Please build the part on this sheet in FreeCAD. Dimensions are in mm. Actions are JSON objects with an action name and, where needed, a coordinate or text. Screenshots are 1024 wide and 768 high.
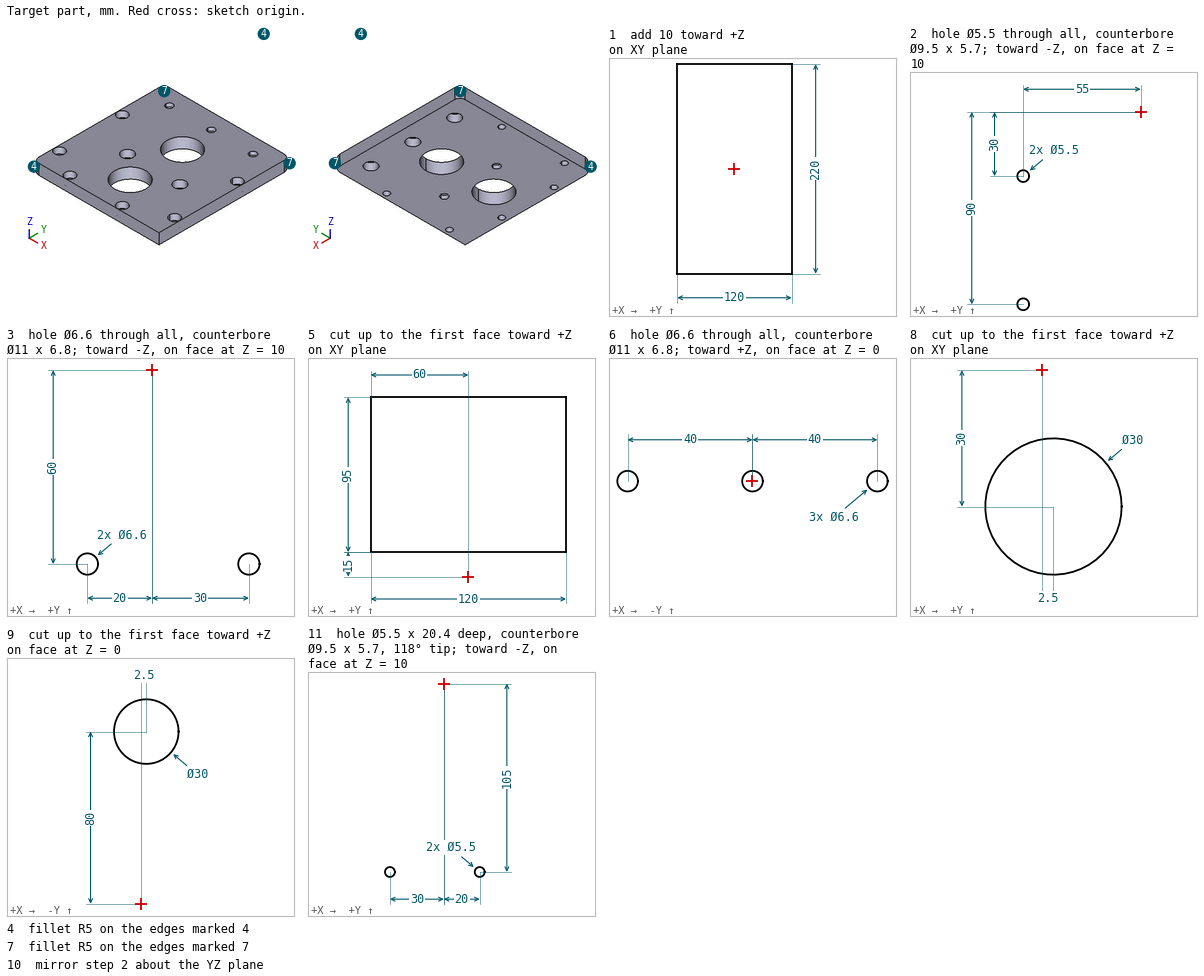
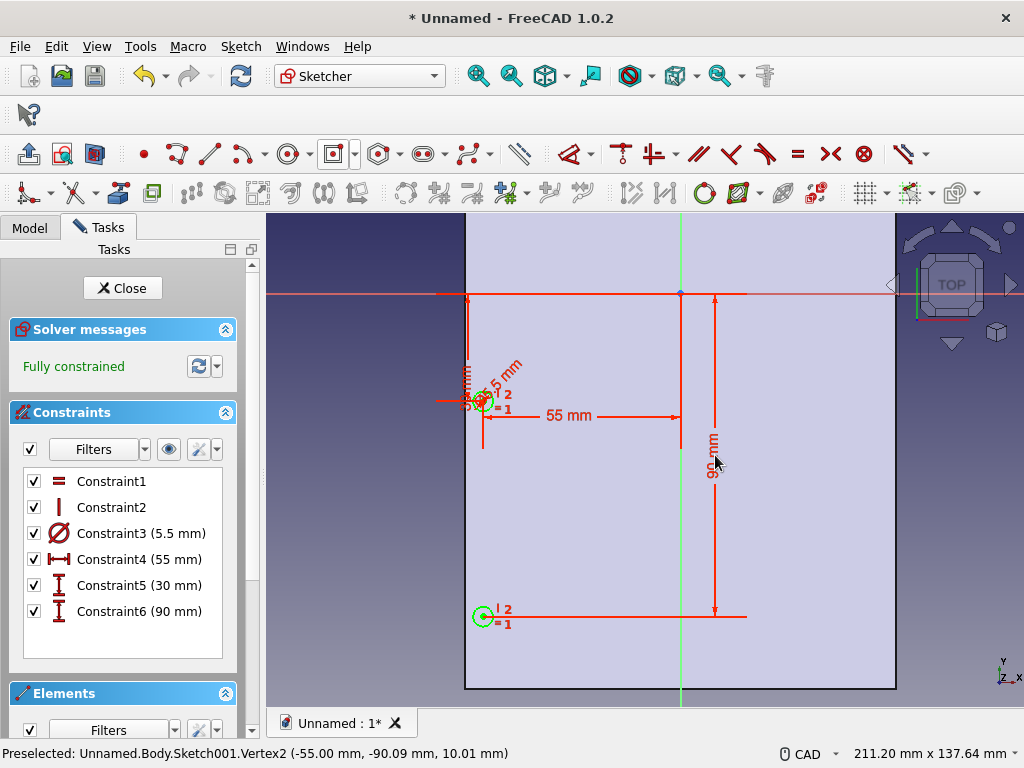
{"action": "left_click", "coordinate": [123, 288]}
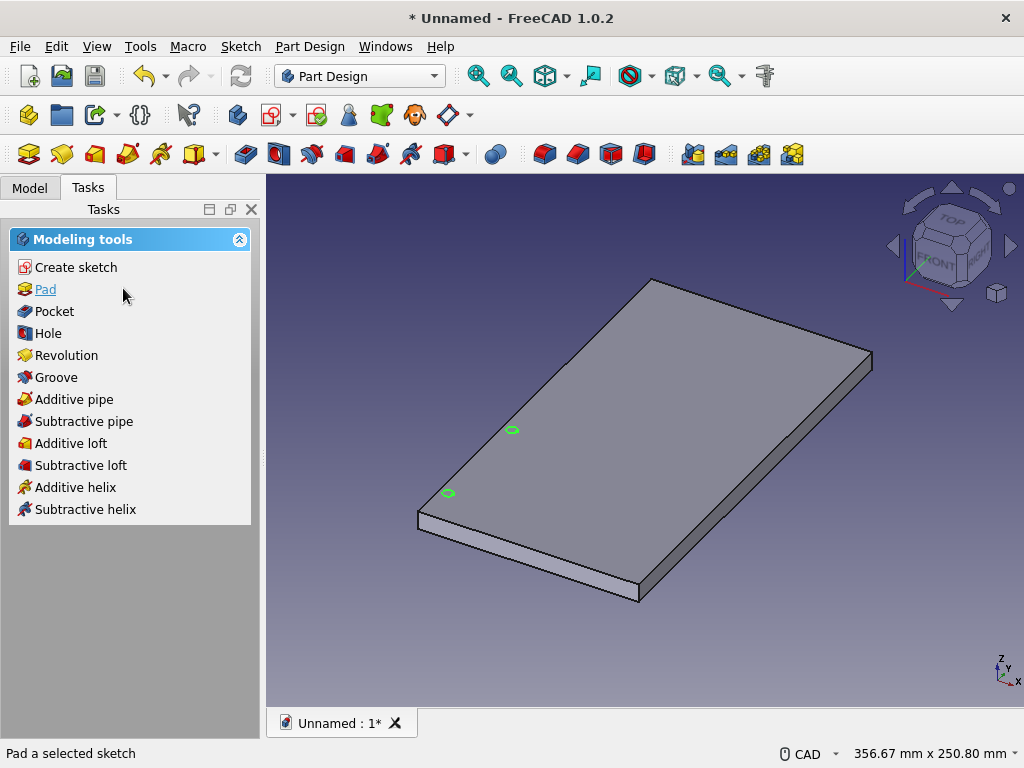
{"action": "left_click", "coordinate": [279, 154]}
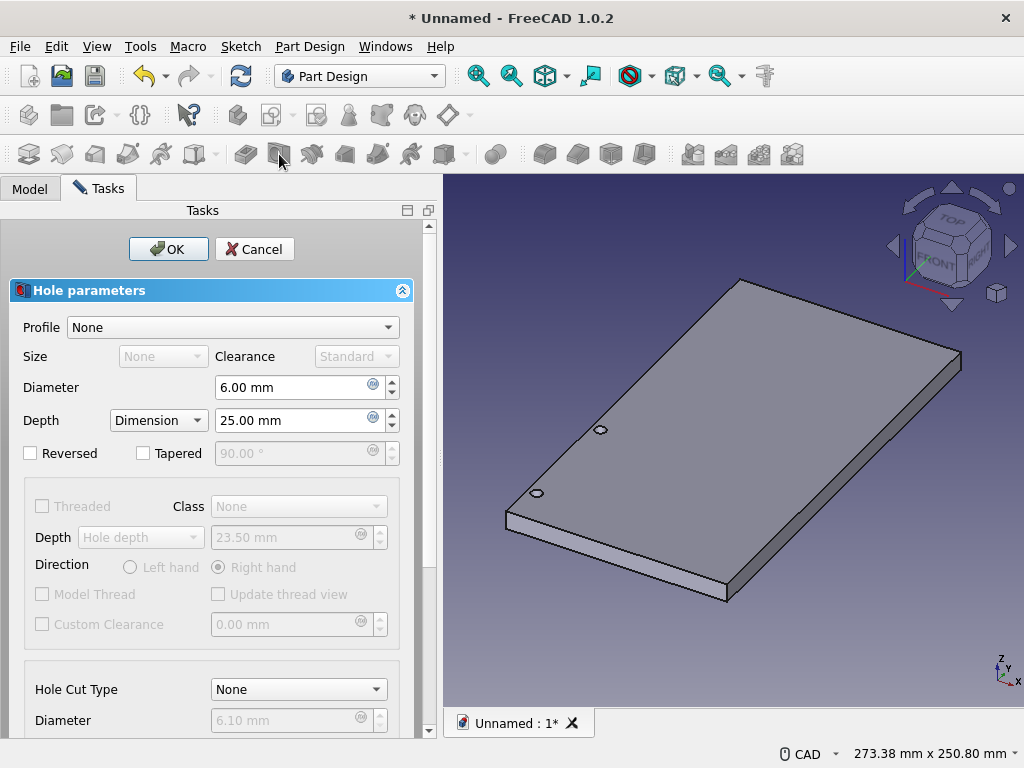
{"action": "triple_click", "coordinate": [300, 388]}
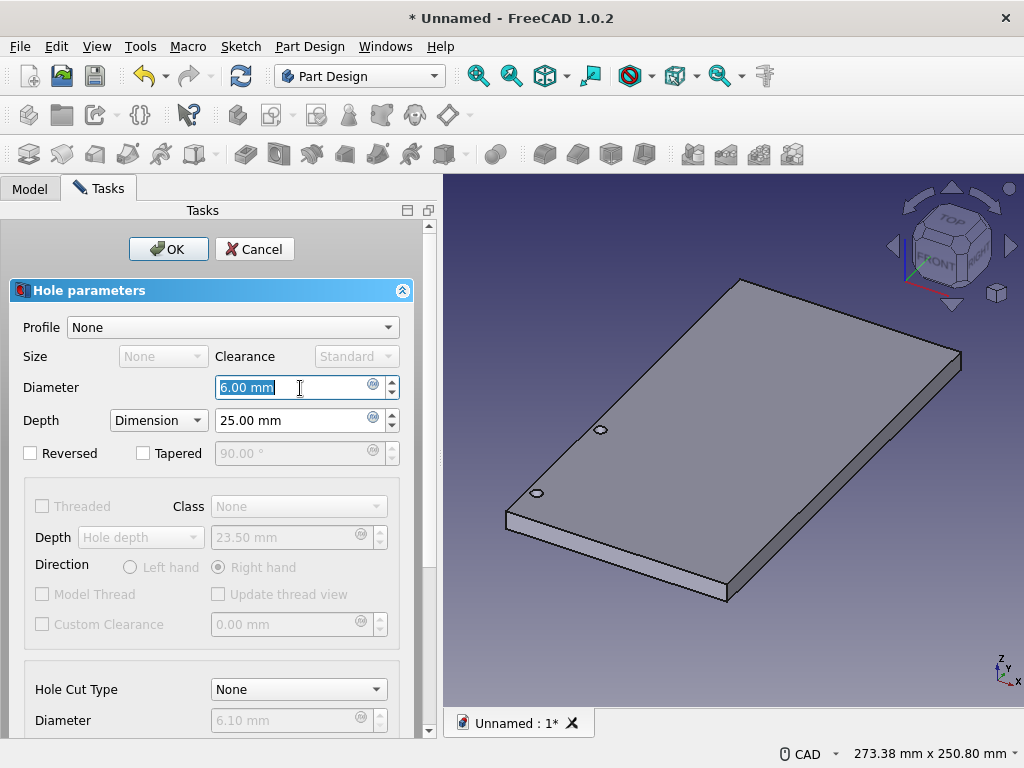
{"action": "type", "text": "5.5"}
{"action": "key", "text": "Tab"}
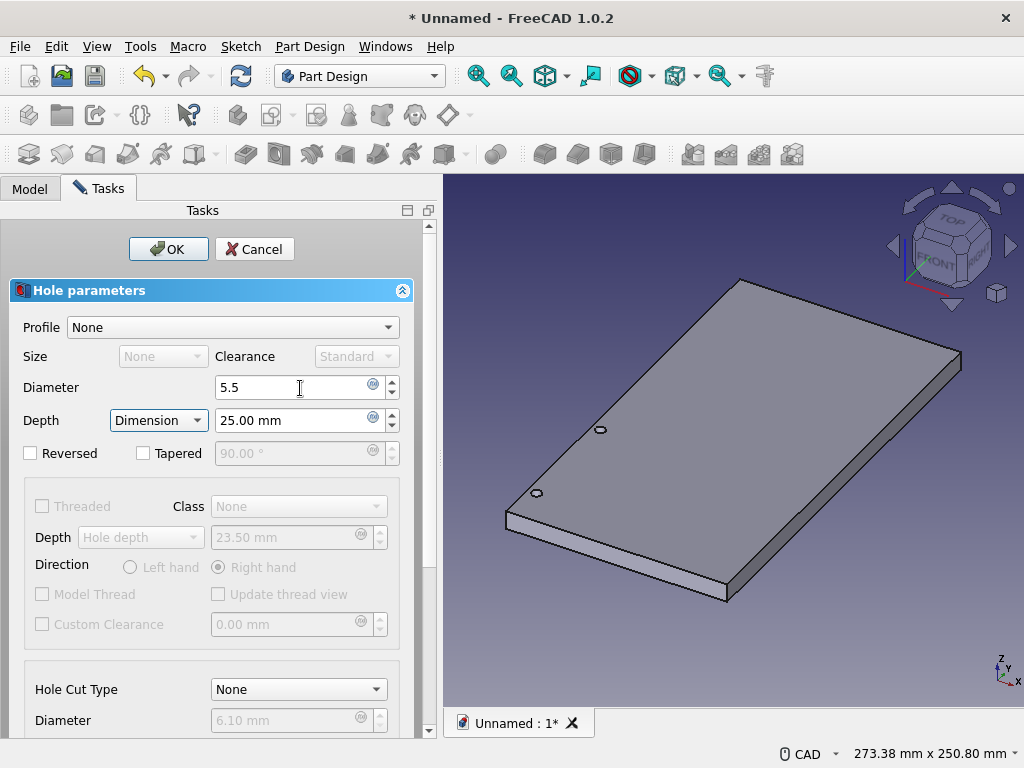
{"action": "left_click", "coordinate": [160, 420]}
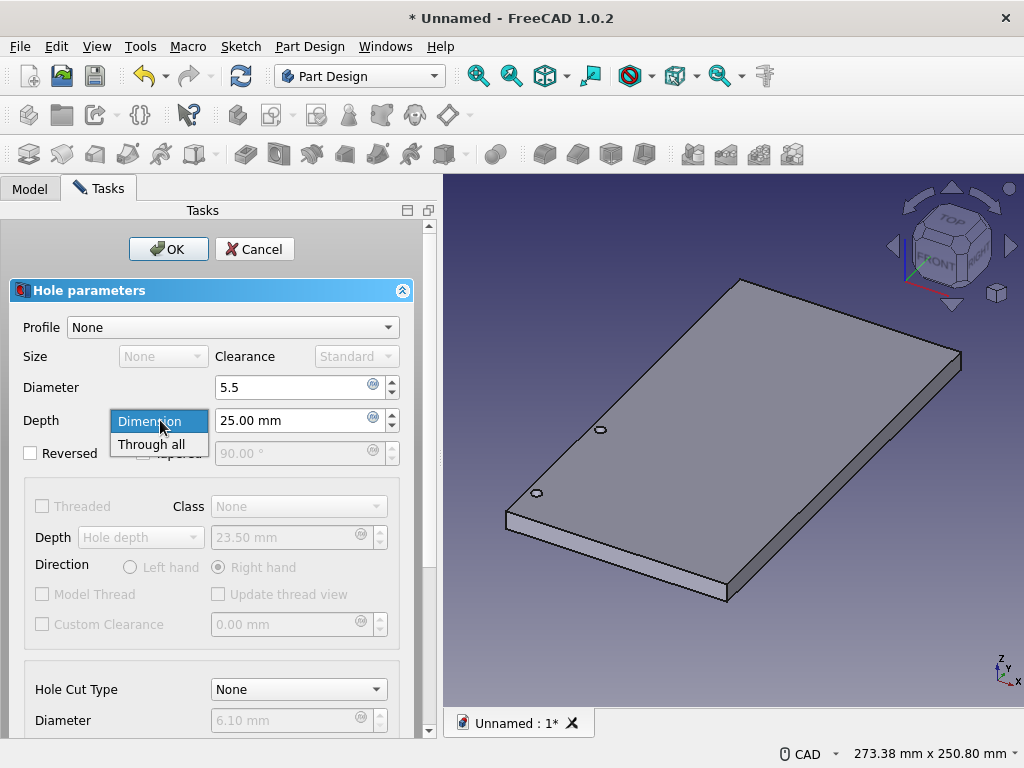
{"action": "left_click", "coordinate": [158, 444]}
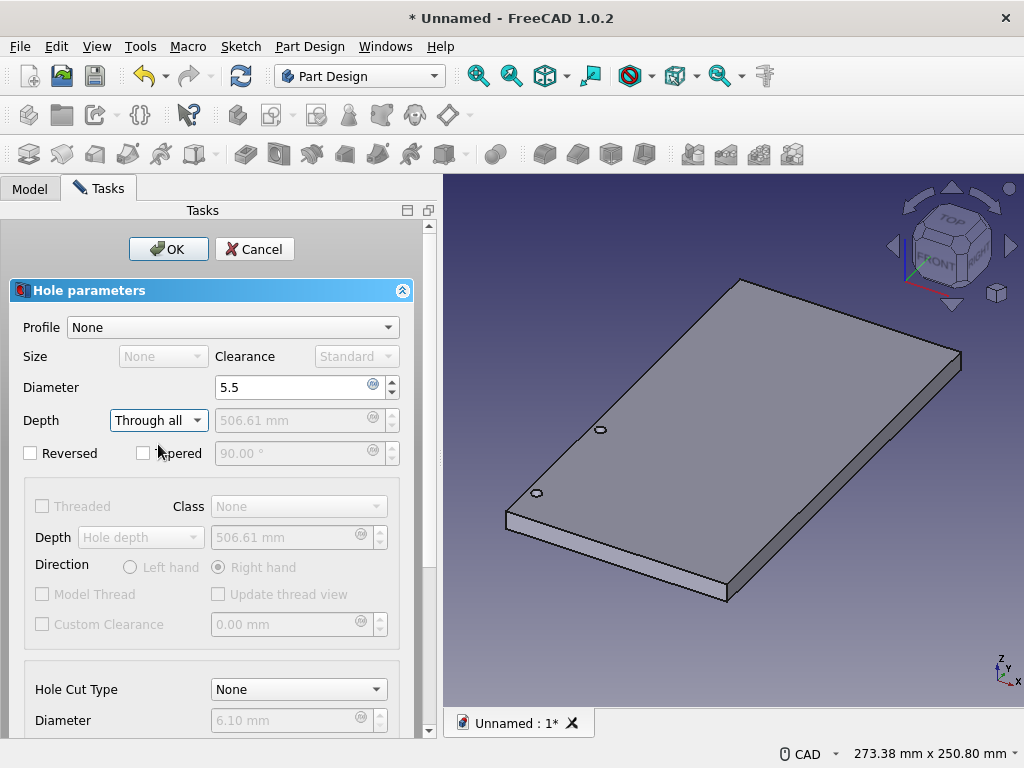
{"action": "left_click", "coordinate": [300, 690]}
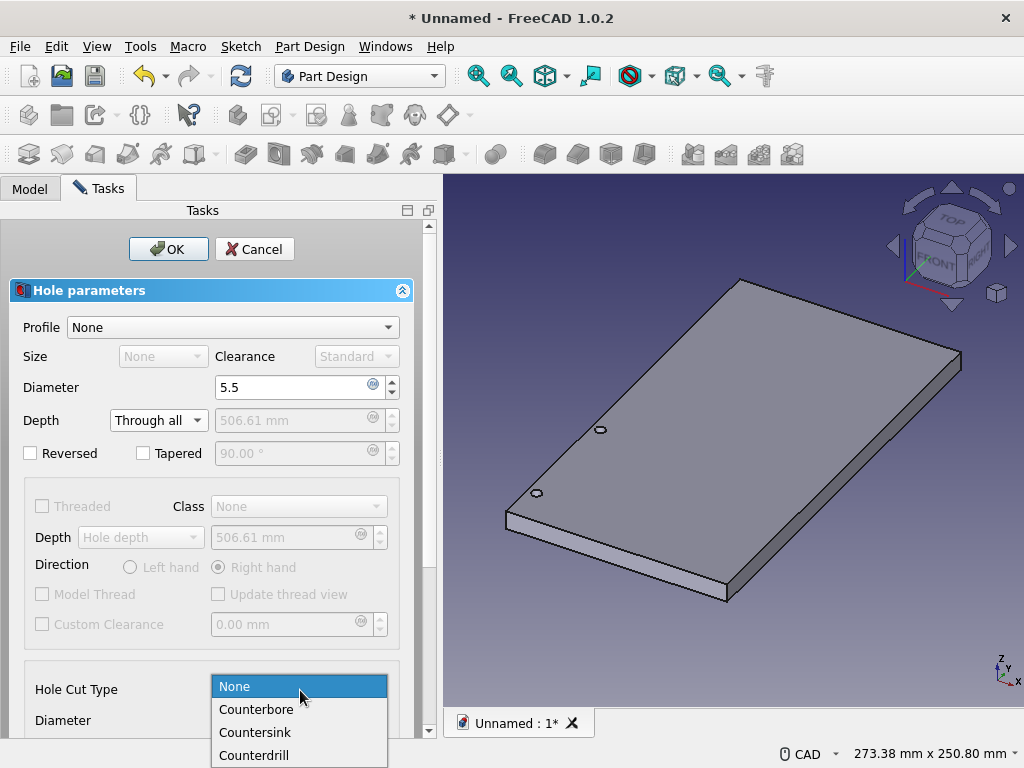
{"action": "left_click", "coordinate": [298, 710]}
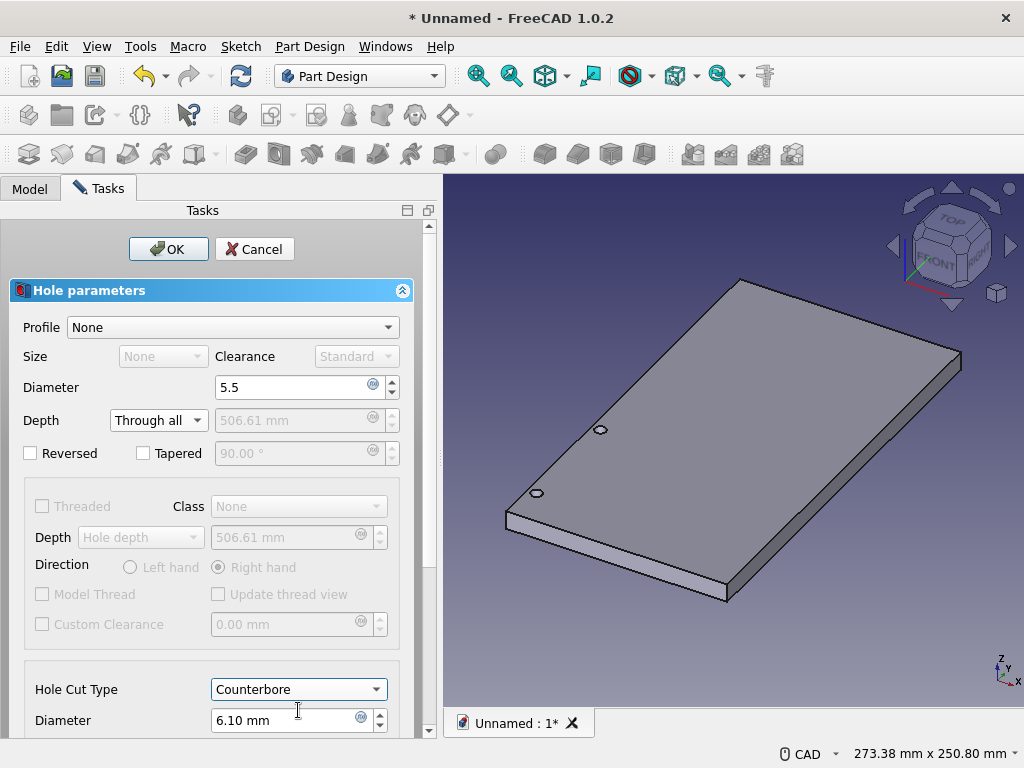
{"action": "triple_click", "coordinate": [292, 720]}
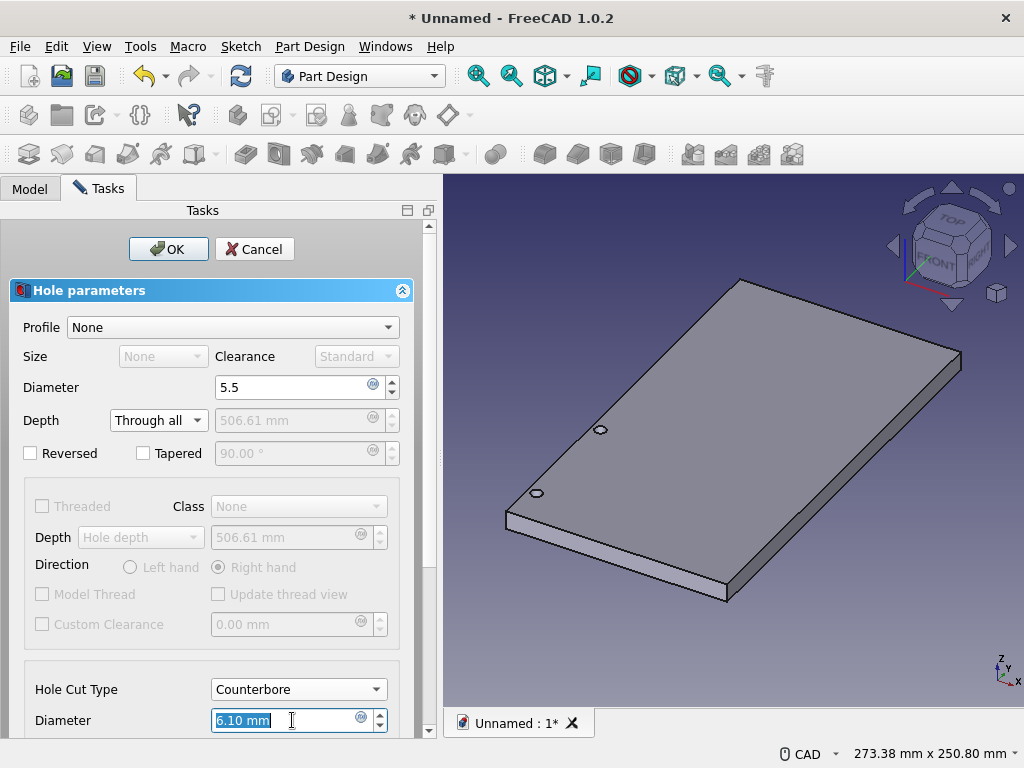
{"action": "type", "text": "9.5"}
{"action": "key", "text": "Tab"}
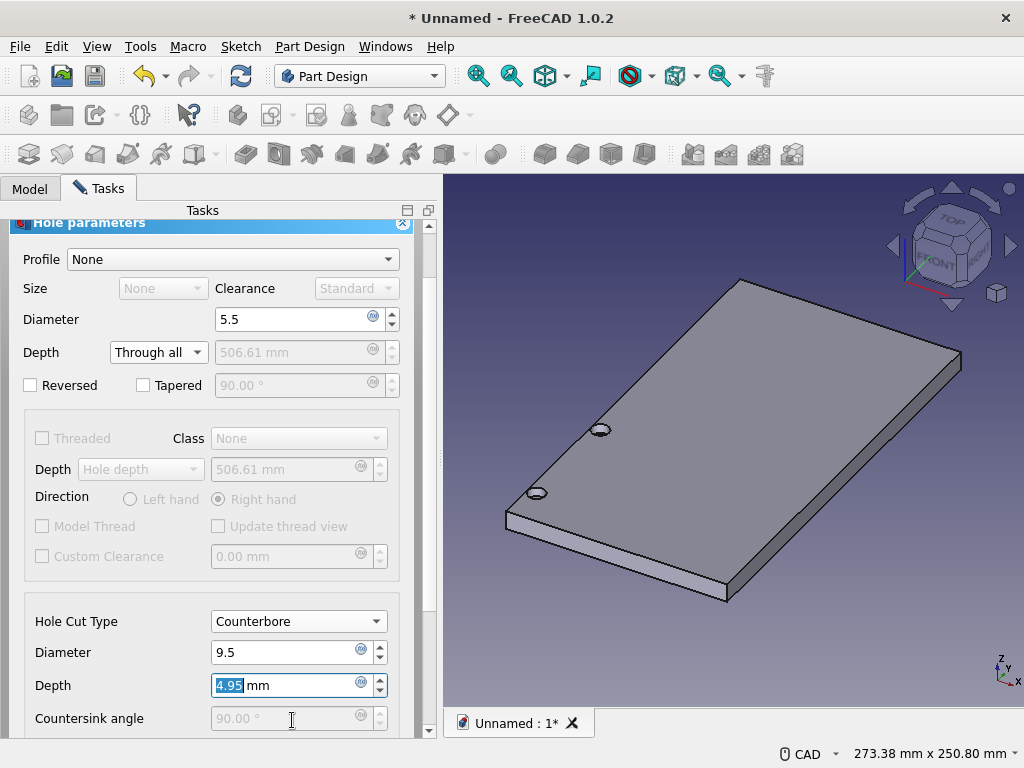
{"action": "type", "text": "5.7"}
{"action": "key", "text": "Tab"}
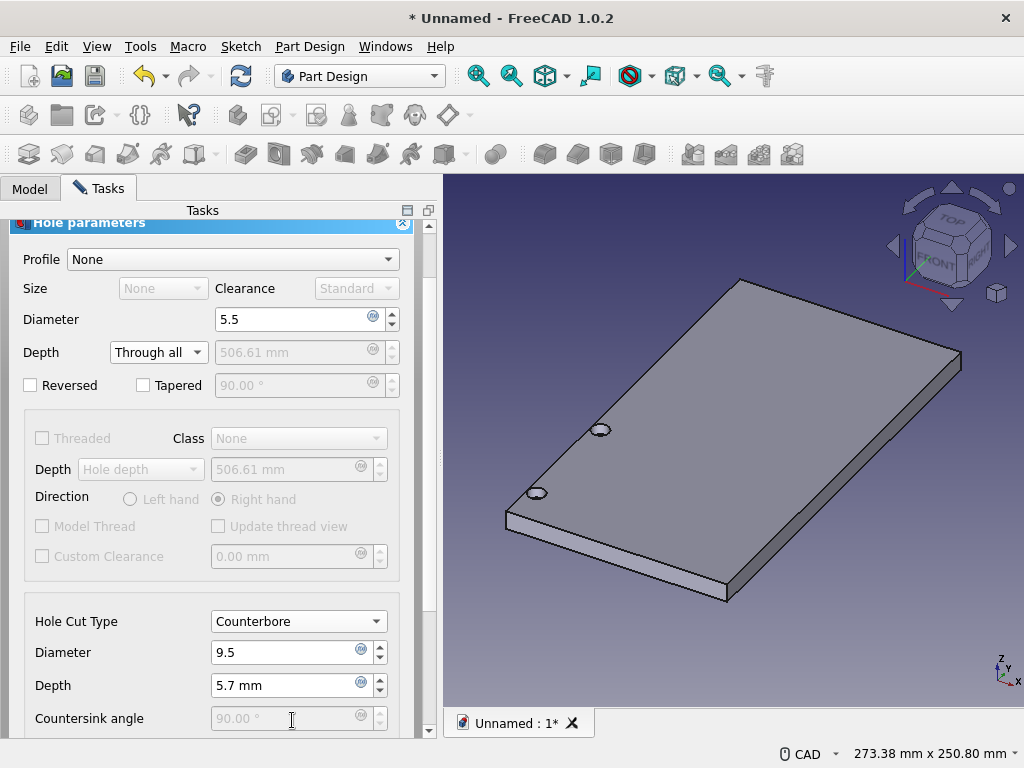
{"action": "scroll", "coordinate": [429, 479], "scroll_direction": "up", "scroll_amount": 2}